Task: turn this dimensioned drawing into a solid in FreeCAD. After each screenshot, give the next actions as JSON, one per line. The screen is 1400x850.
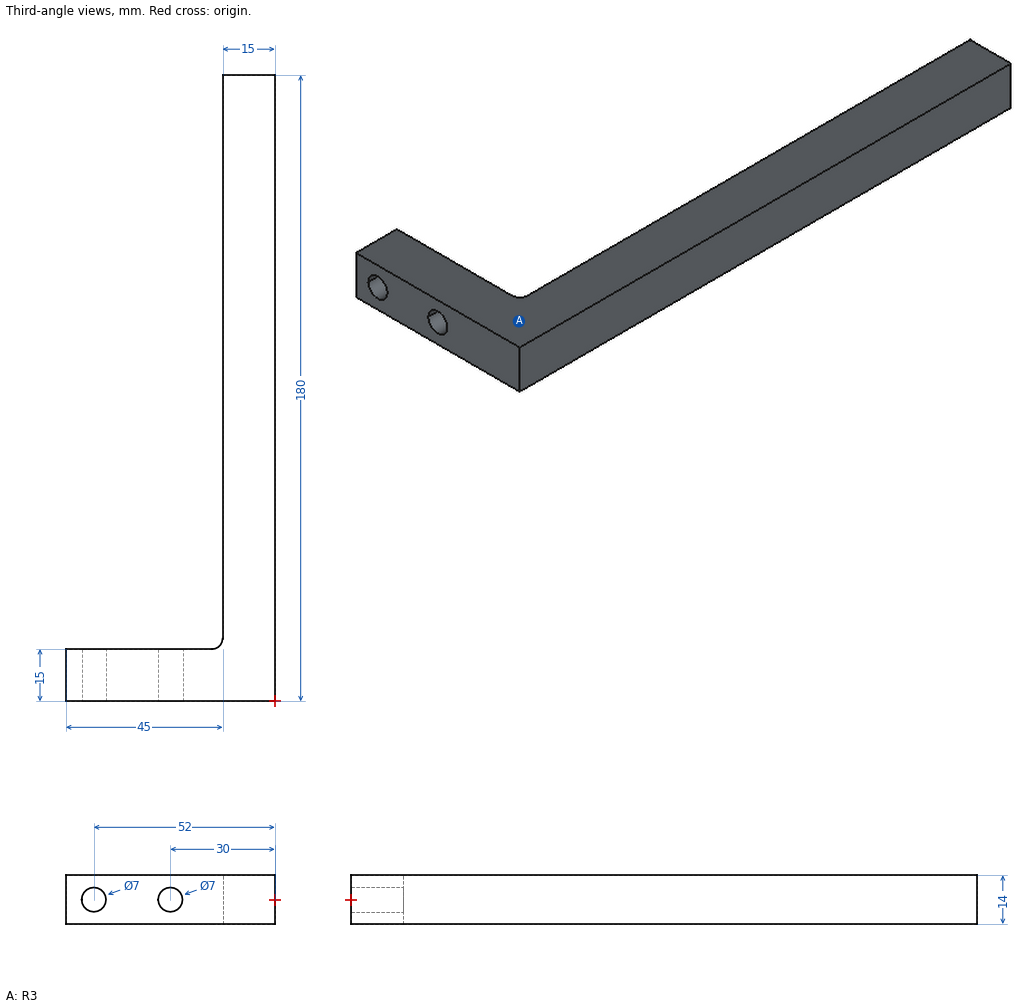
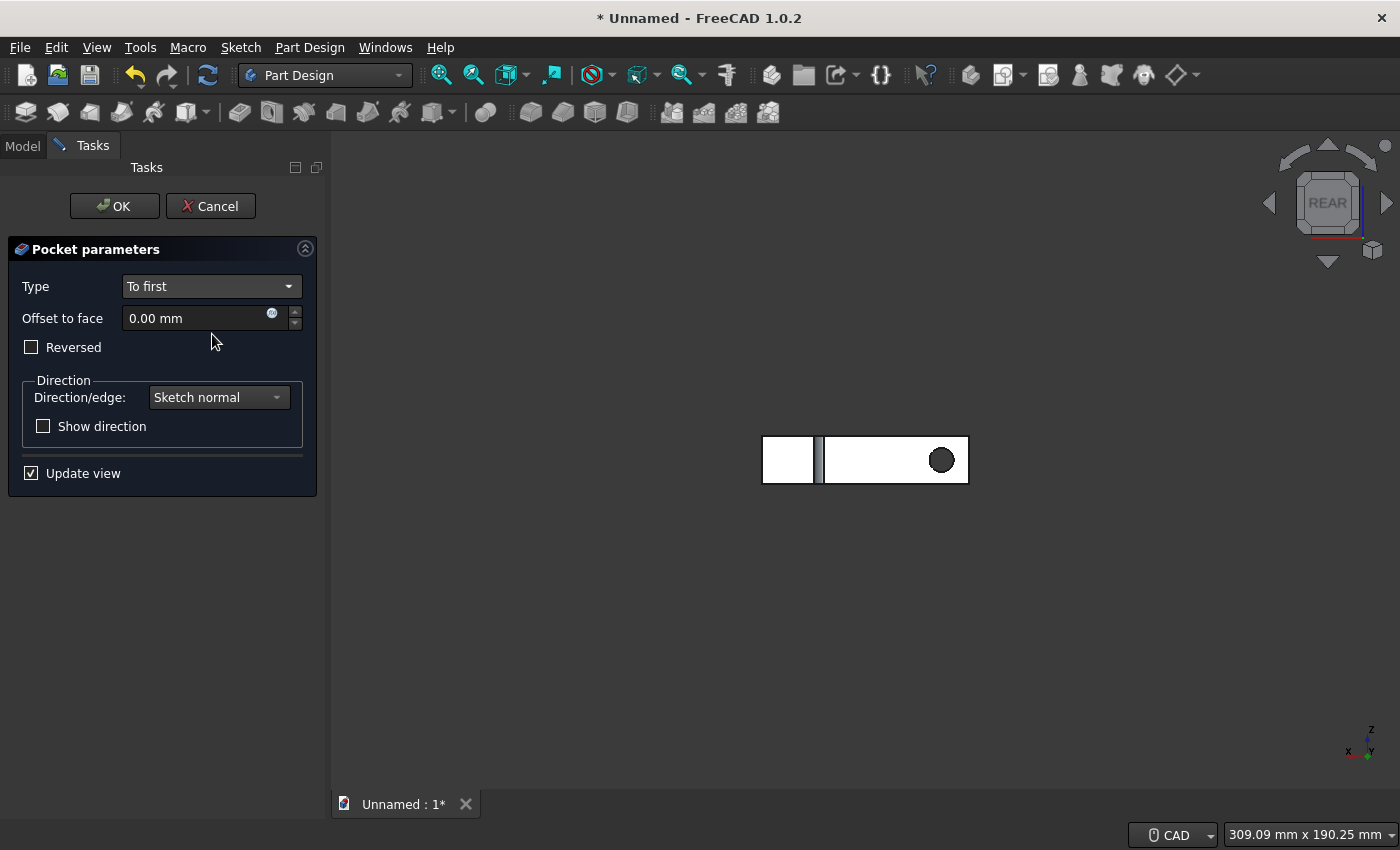
{"action": "left_click", "coordinate": [115, 206]}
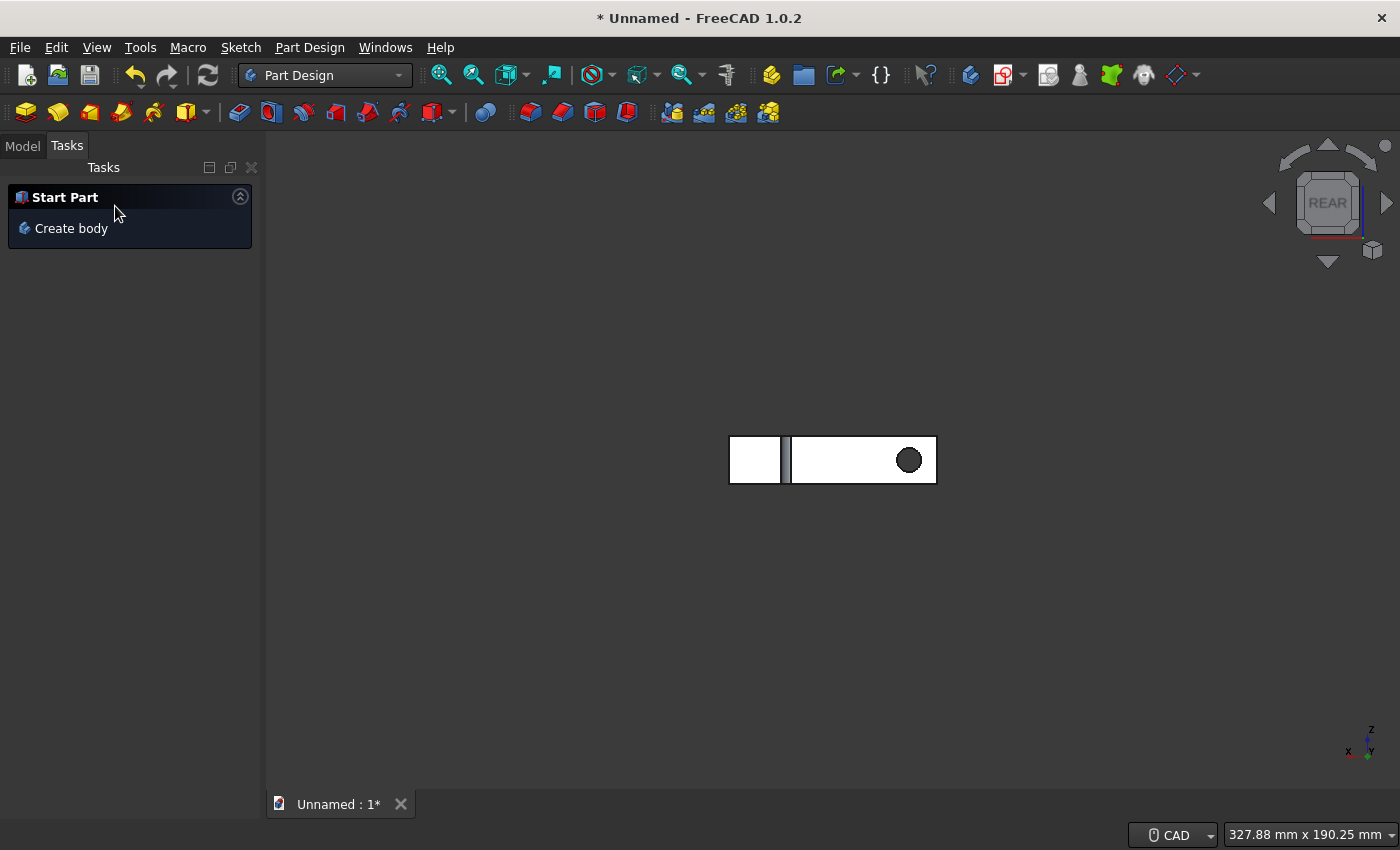
{"action": "left_click", "coordinate": [442, 76]}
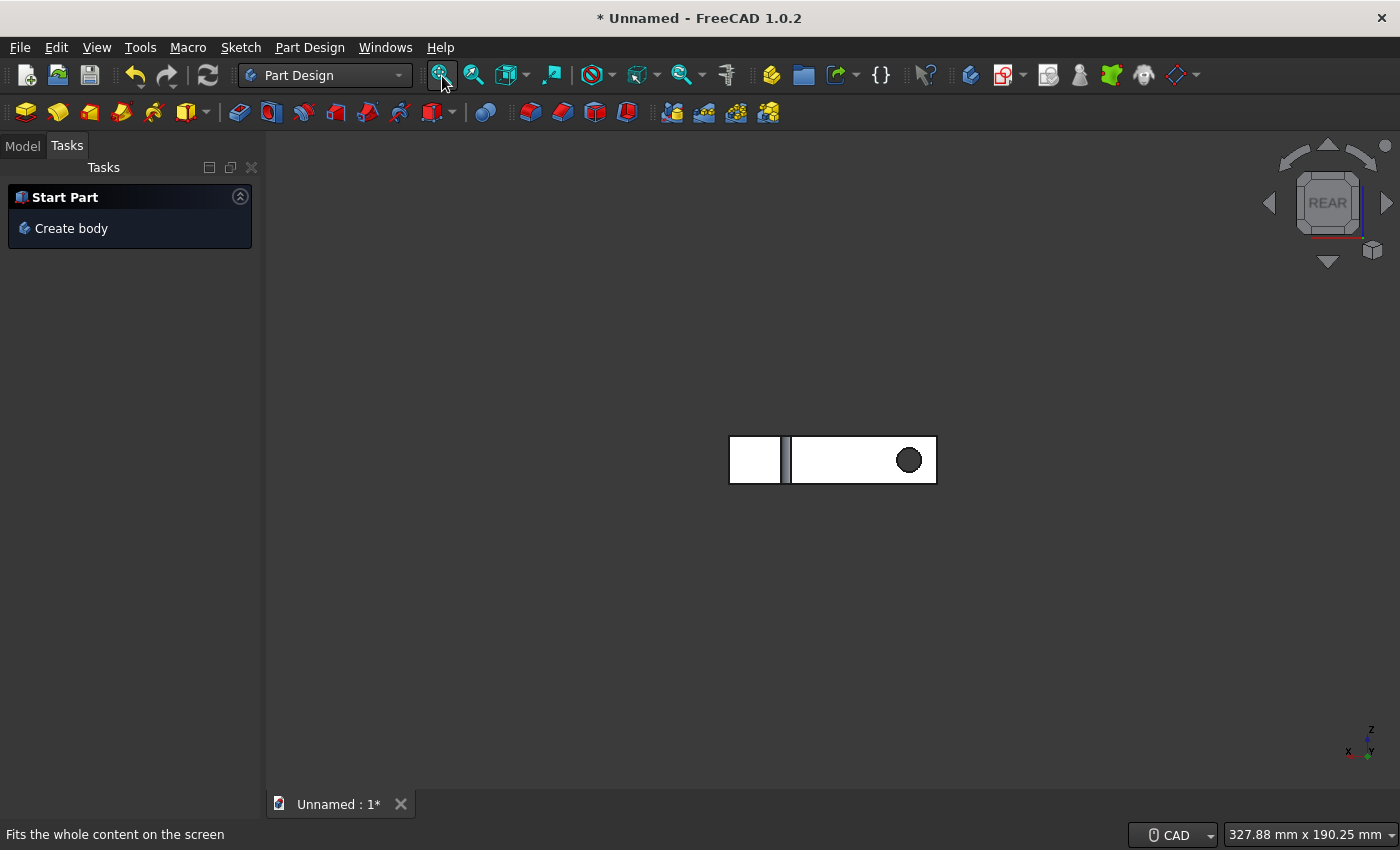
{"action": "left_click", "coordinate": [823, 459]}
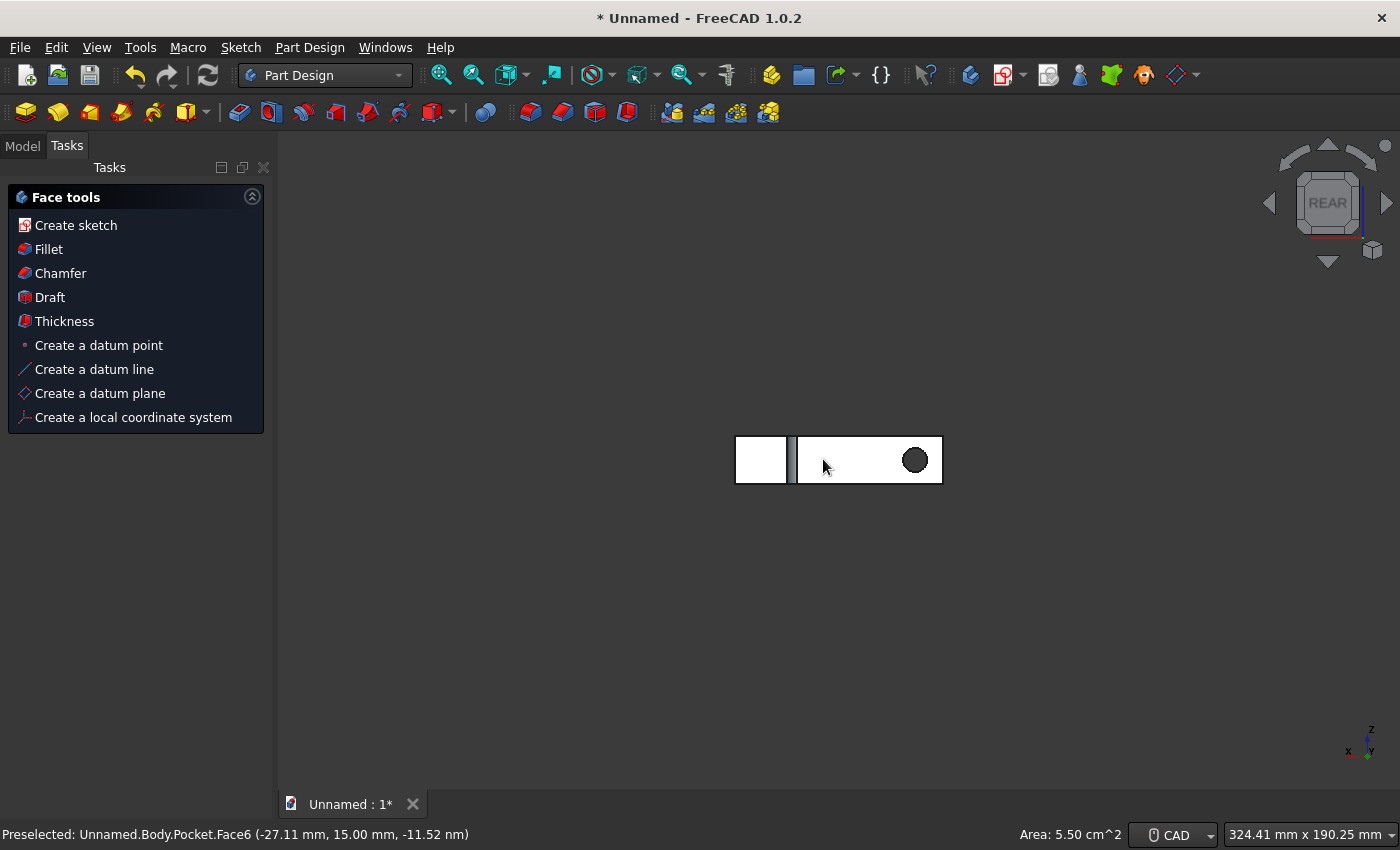
{"action": "left_click", "coordinate": [1004, 76]}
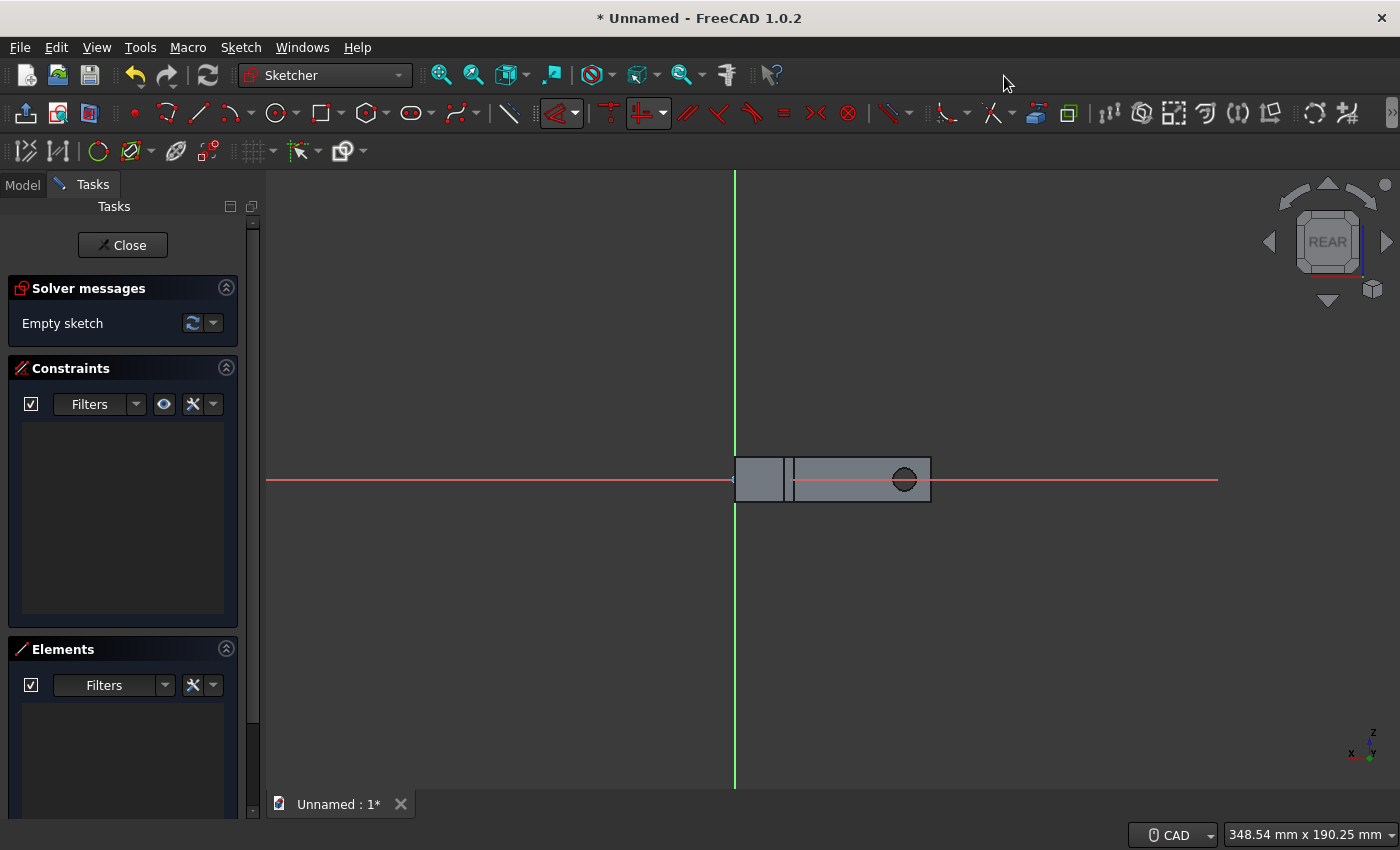
{"action": "left_click", "coordinate": [90, 114]}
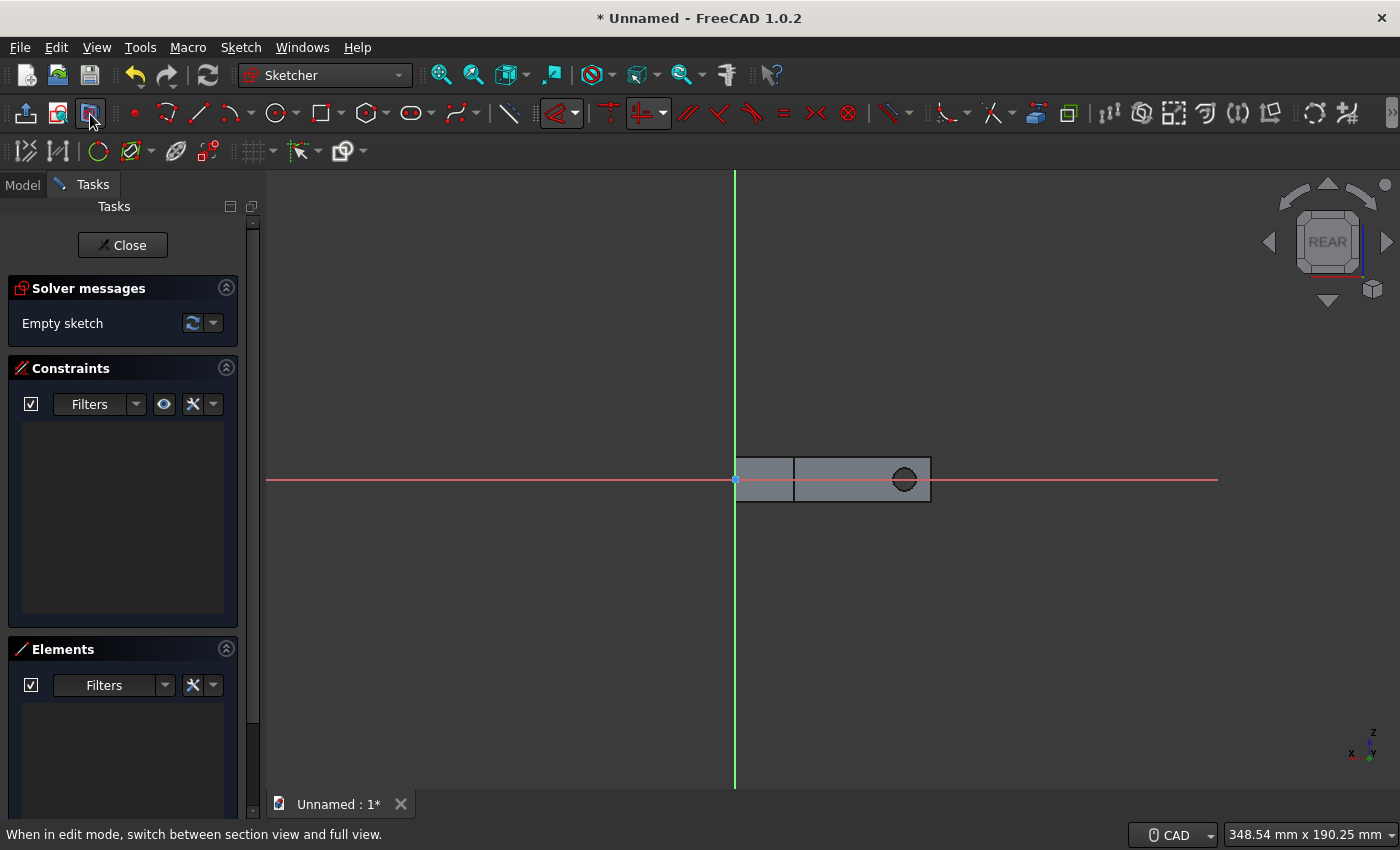
{"action": "scroll", "coordinate": [837, 480], "scroll_direction": "up", "scroll_amount": 14}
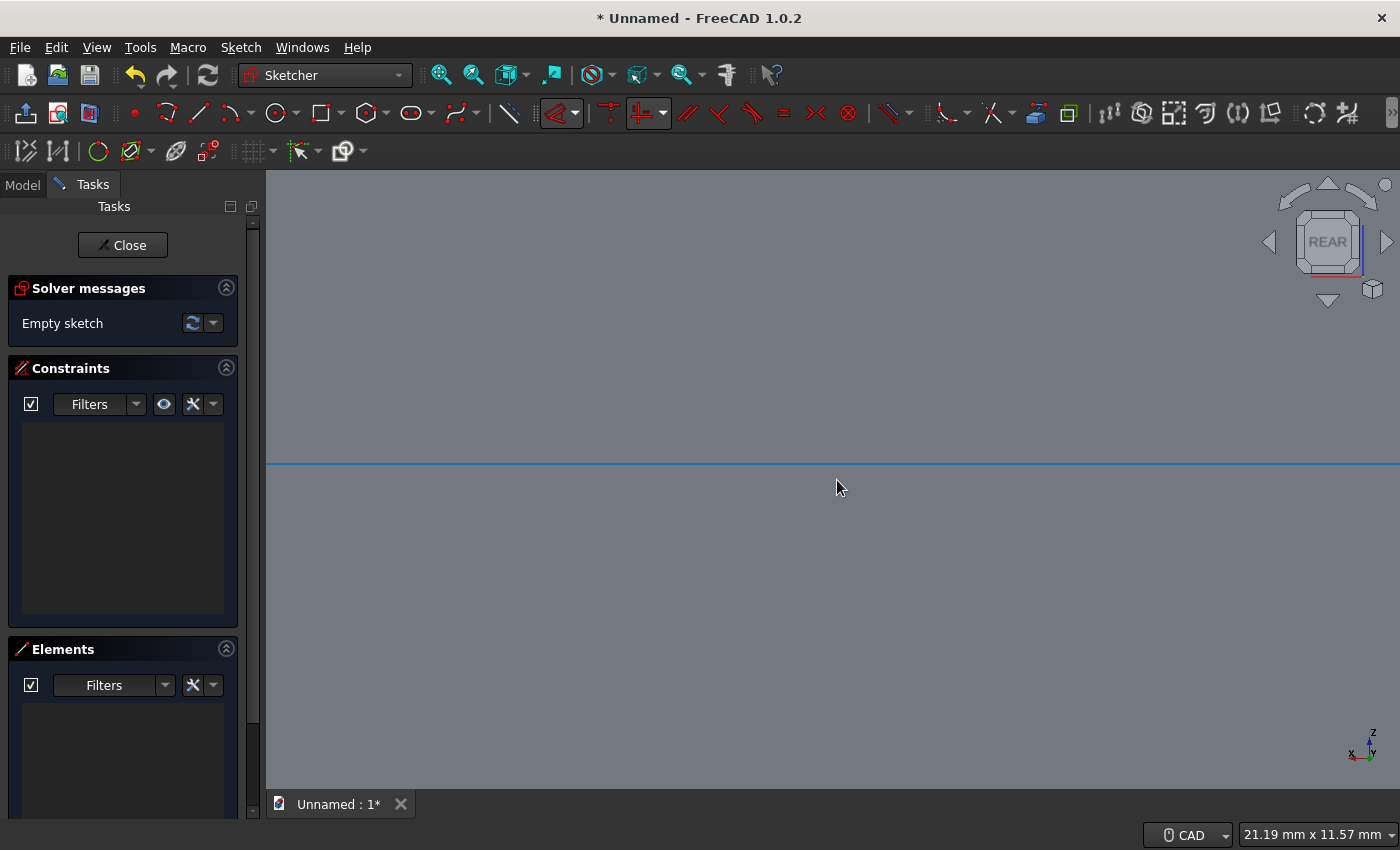
{"action": "left_click", "coordinate": [276, 114]}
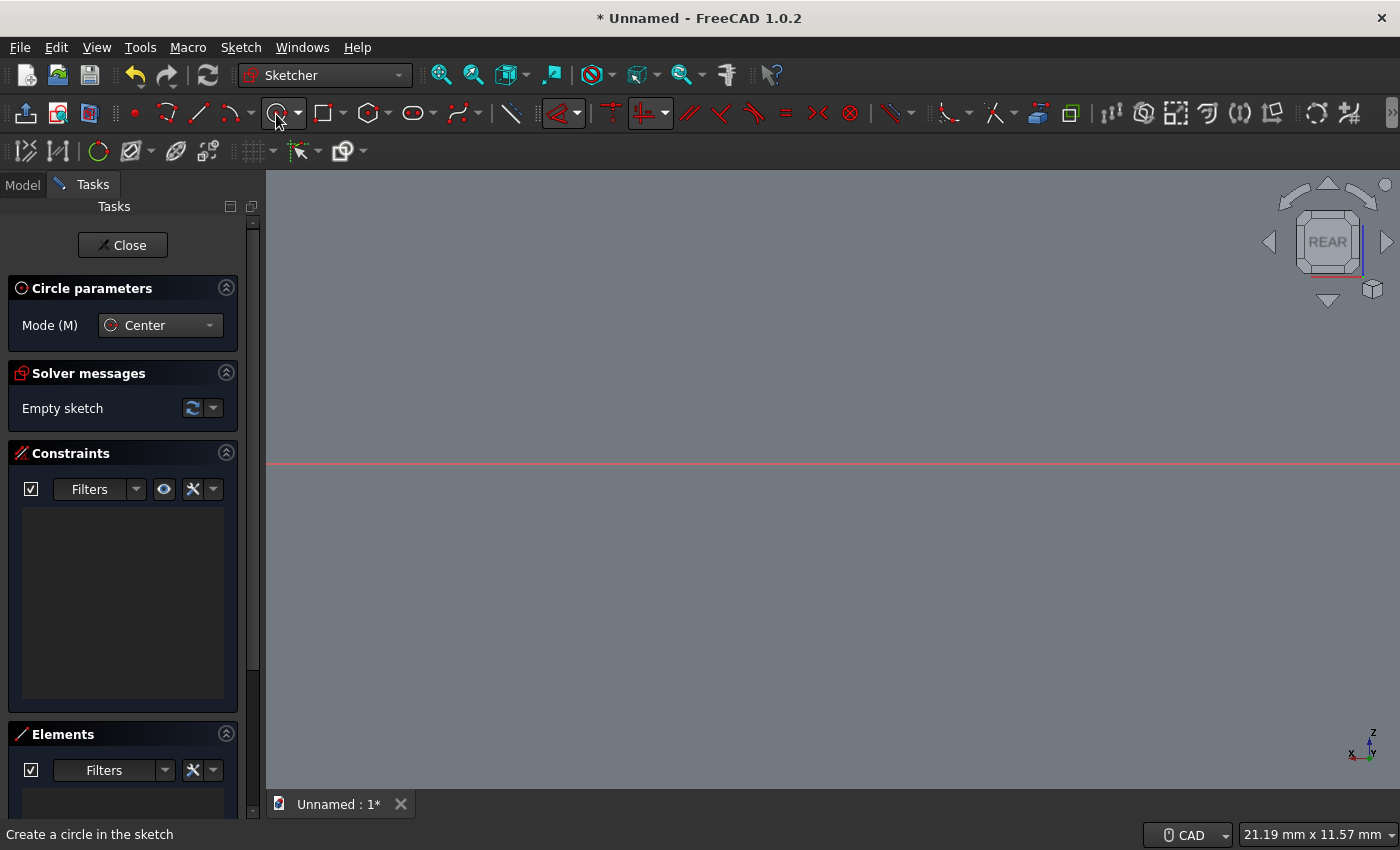
{"action": "left_click", "coordinate": [763, 464]}
{"action": "mouse_move", "coordinate": [896, 332]}